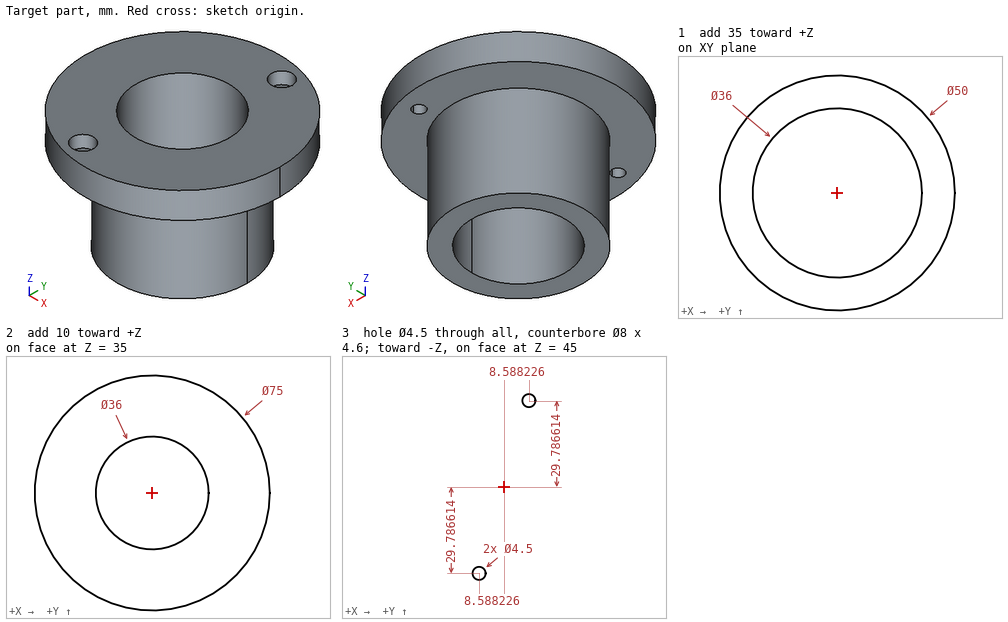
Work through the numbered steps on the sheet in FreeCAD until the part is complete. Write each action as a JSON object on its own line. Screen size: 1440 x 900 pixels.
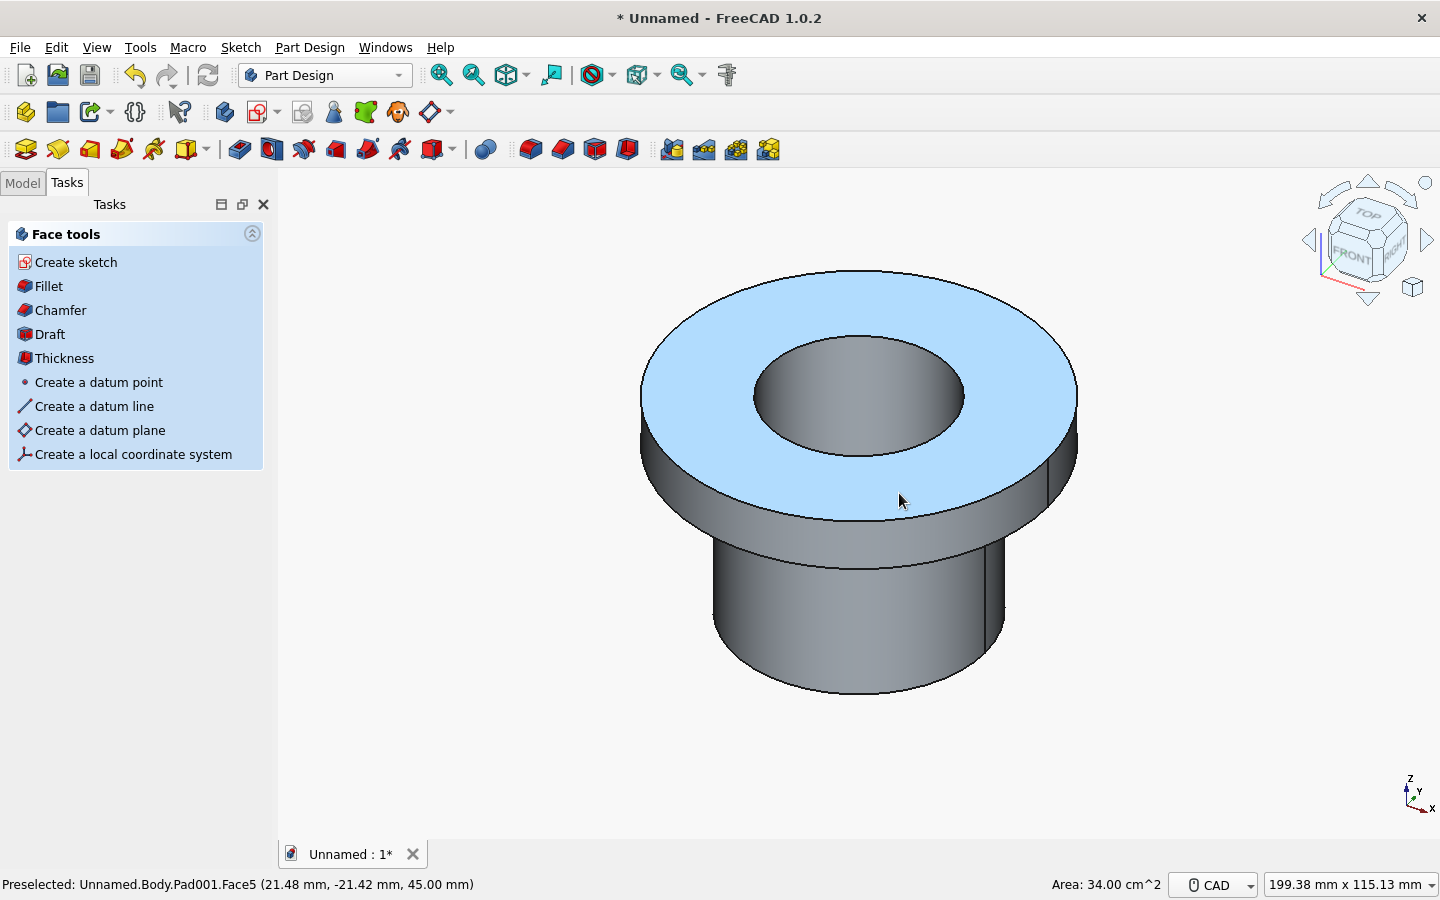
{"action": "left_click", "coordinate": [258, 112]}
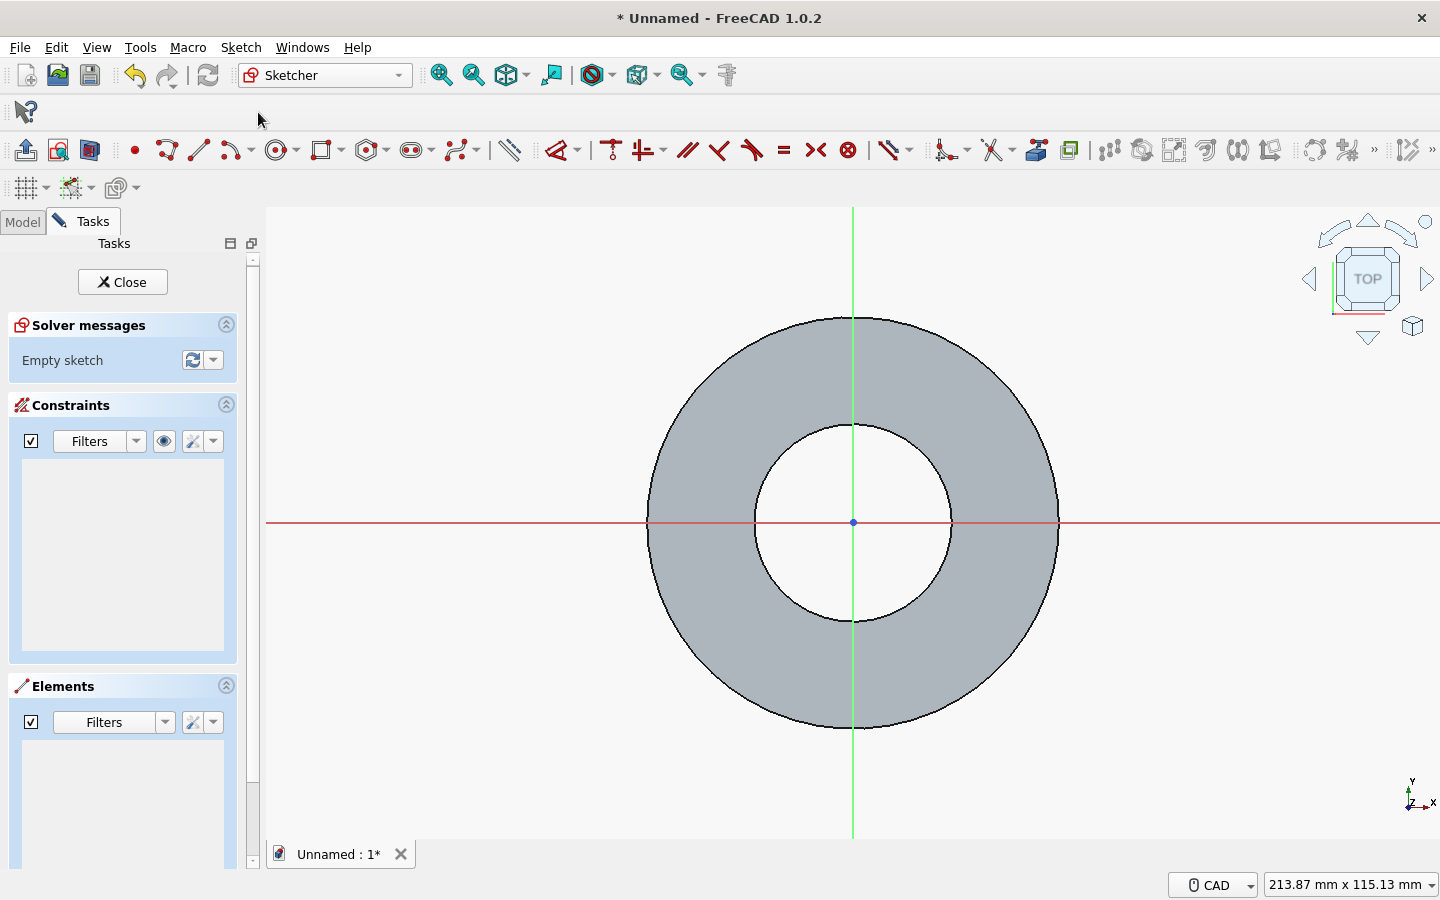
{"action": "key", "text": "g c"}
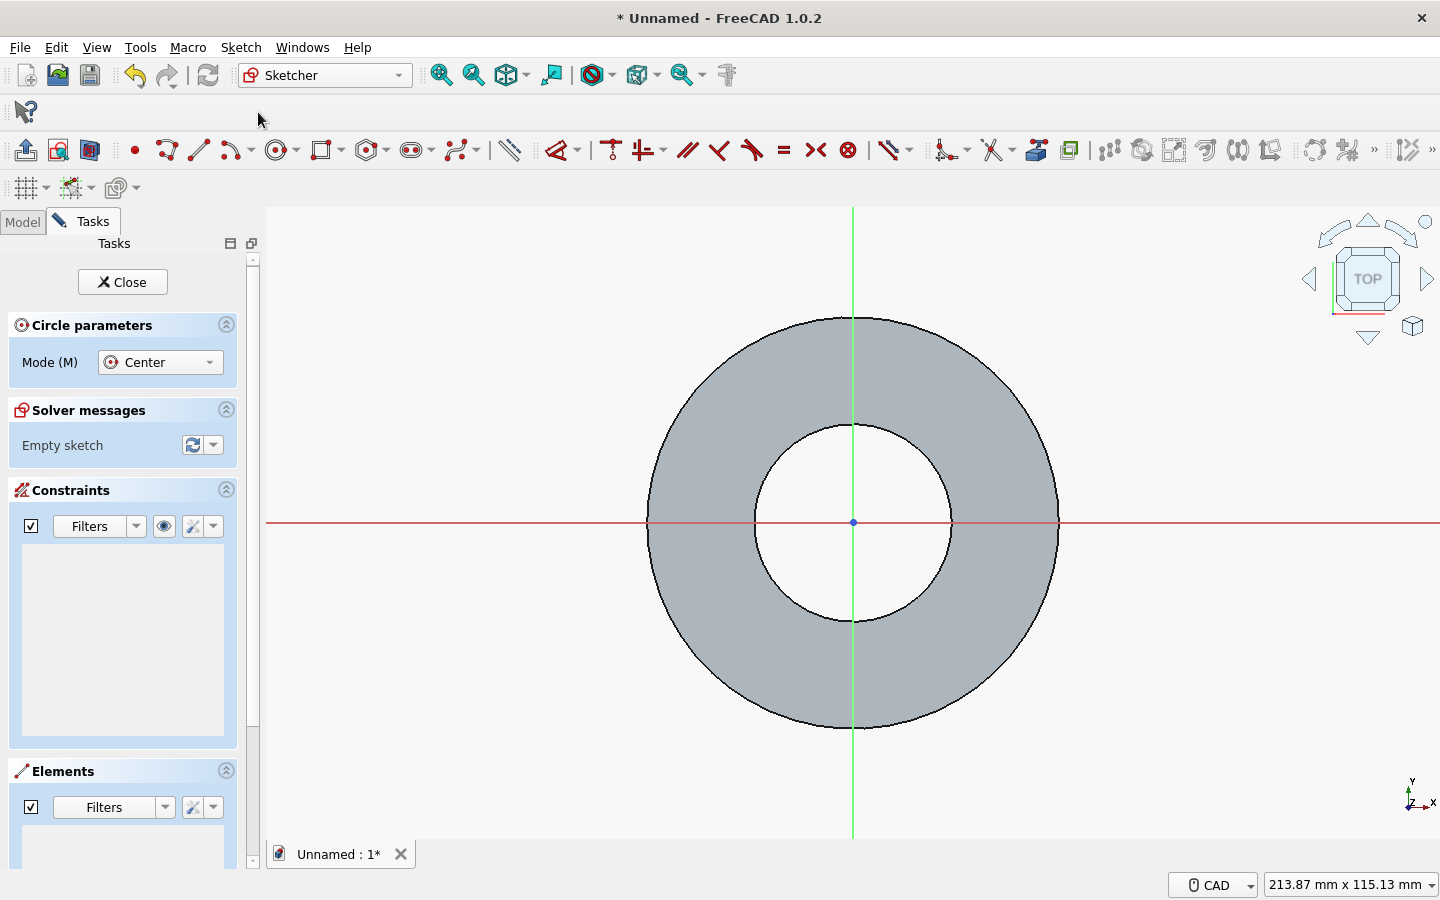
{"action": "scroll", "coordinate": [806, 687], "scroll_direction": "up", "scroll_amount": 4}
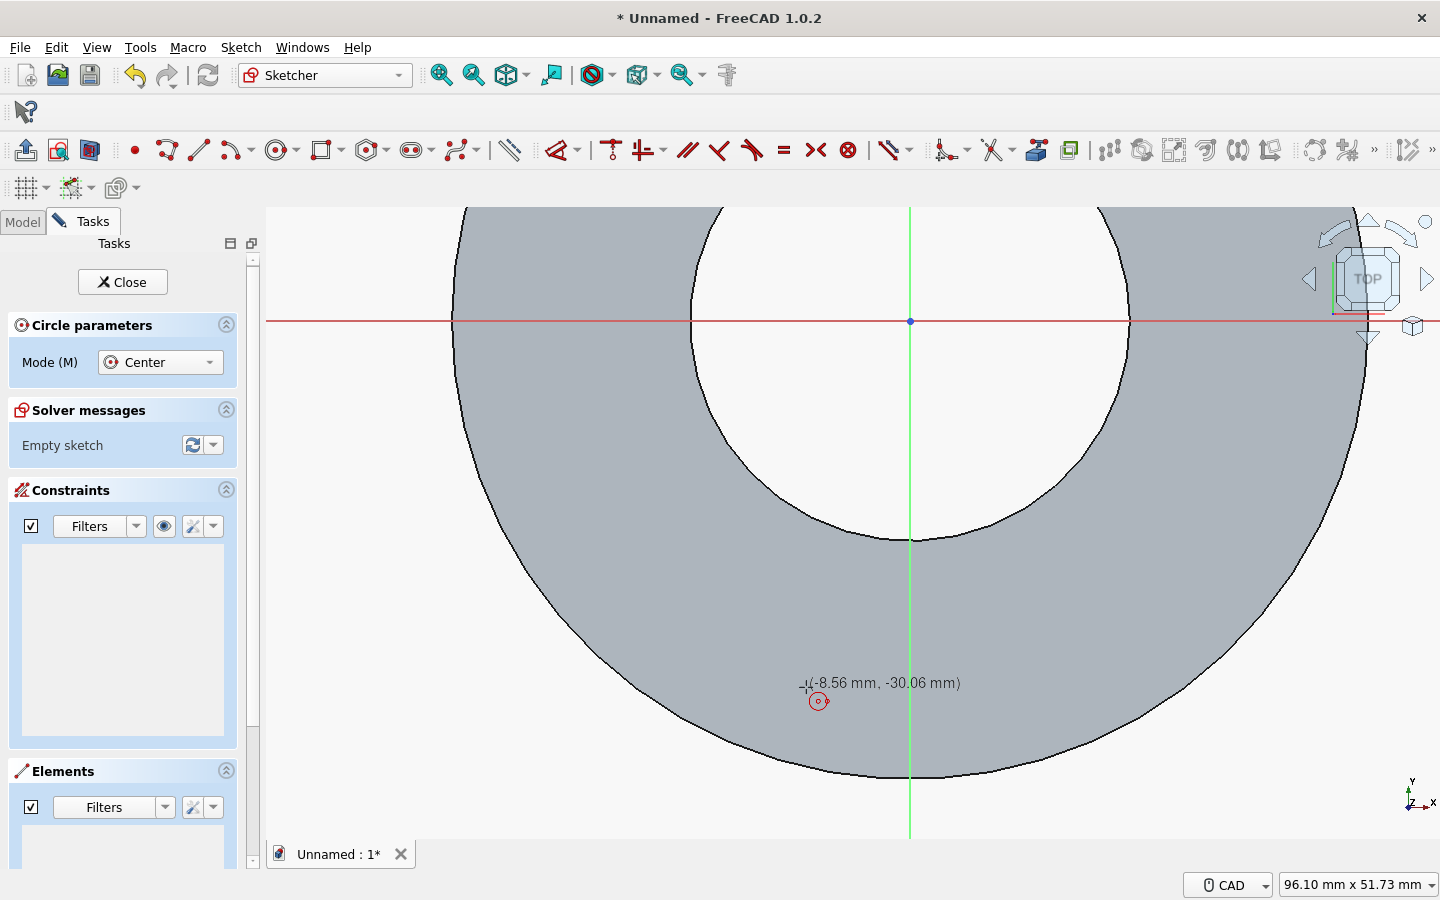
{"action": "left_click", "coordinate": [805, 685]}
{"action": "left_click", "coordinate": [825, 666]}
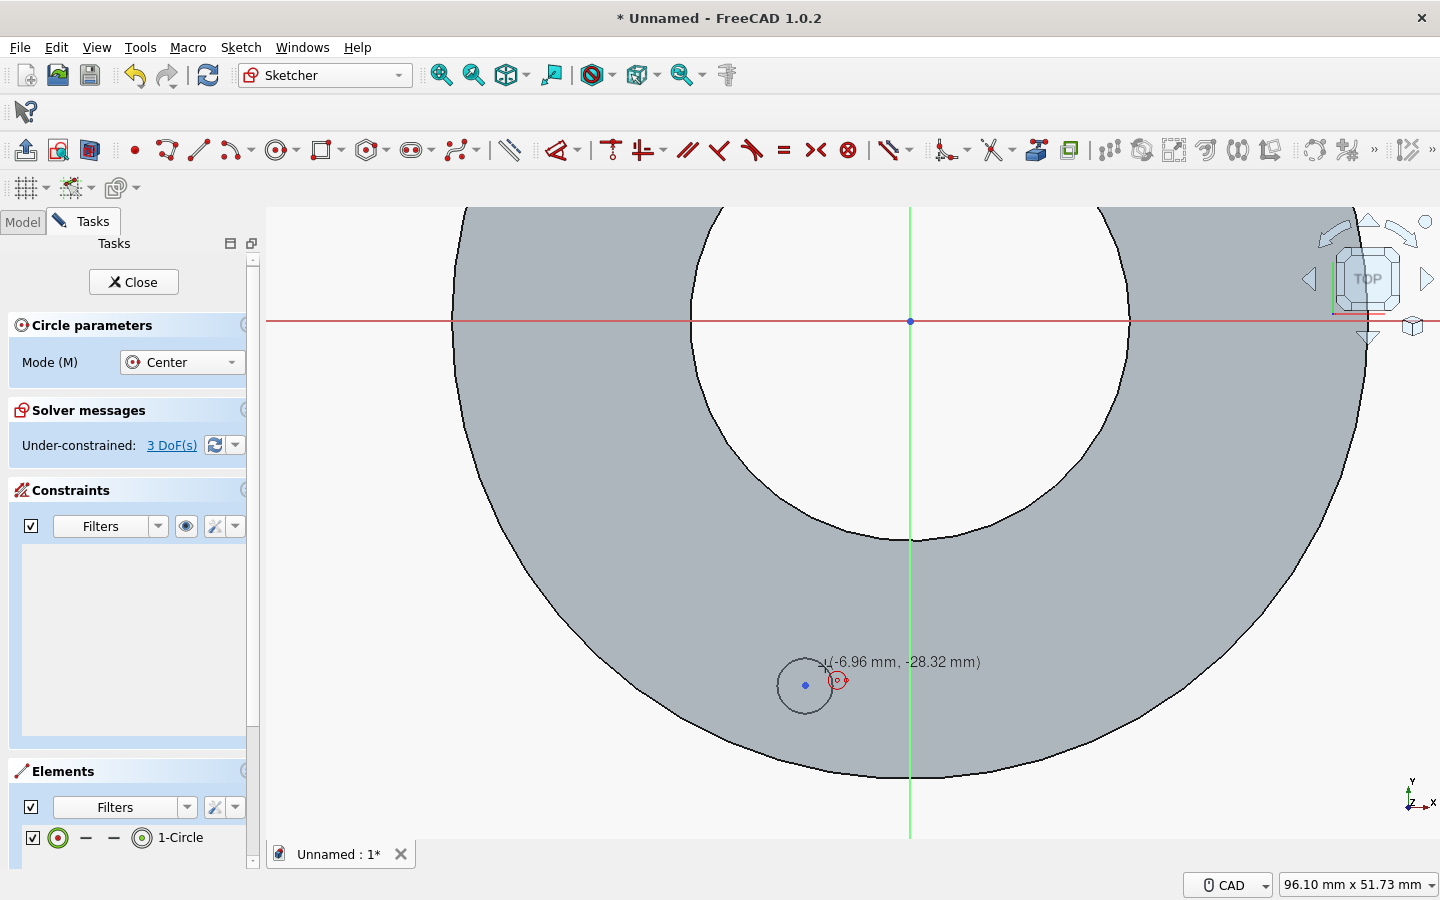
{"action": "scroll", "coordinate": [632, 769], "scroll_direction": "down", "scroll_amount": 3}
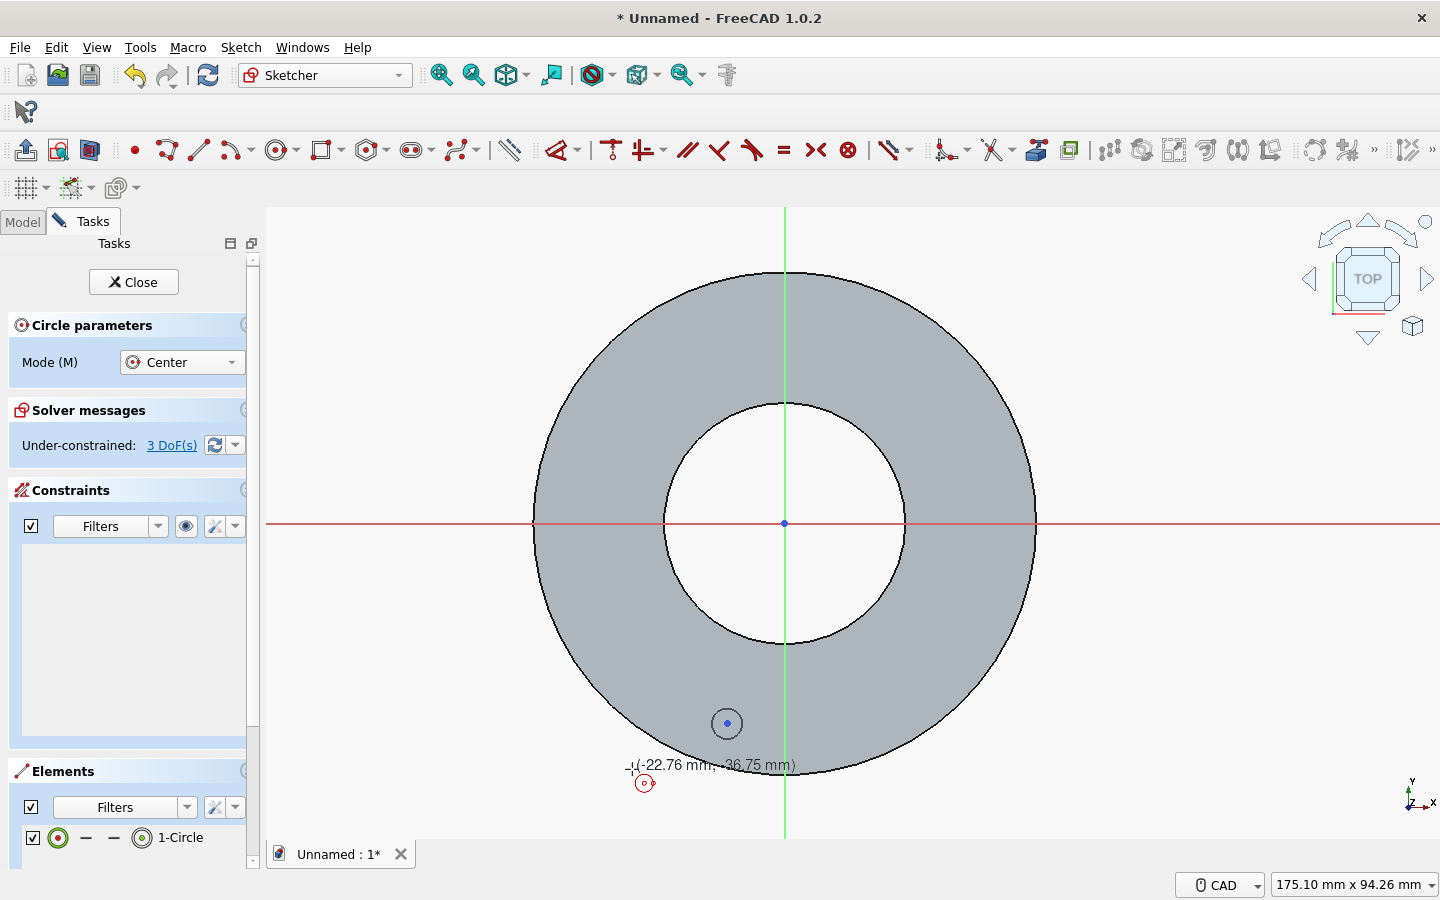
{"action": "scroll", "coordinate": [842, 324], "scroll_direction": "up", "scroll_amount": 3}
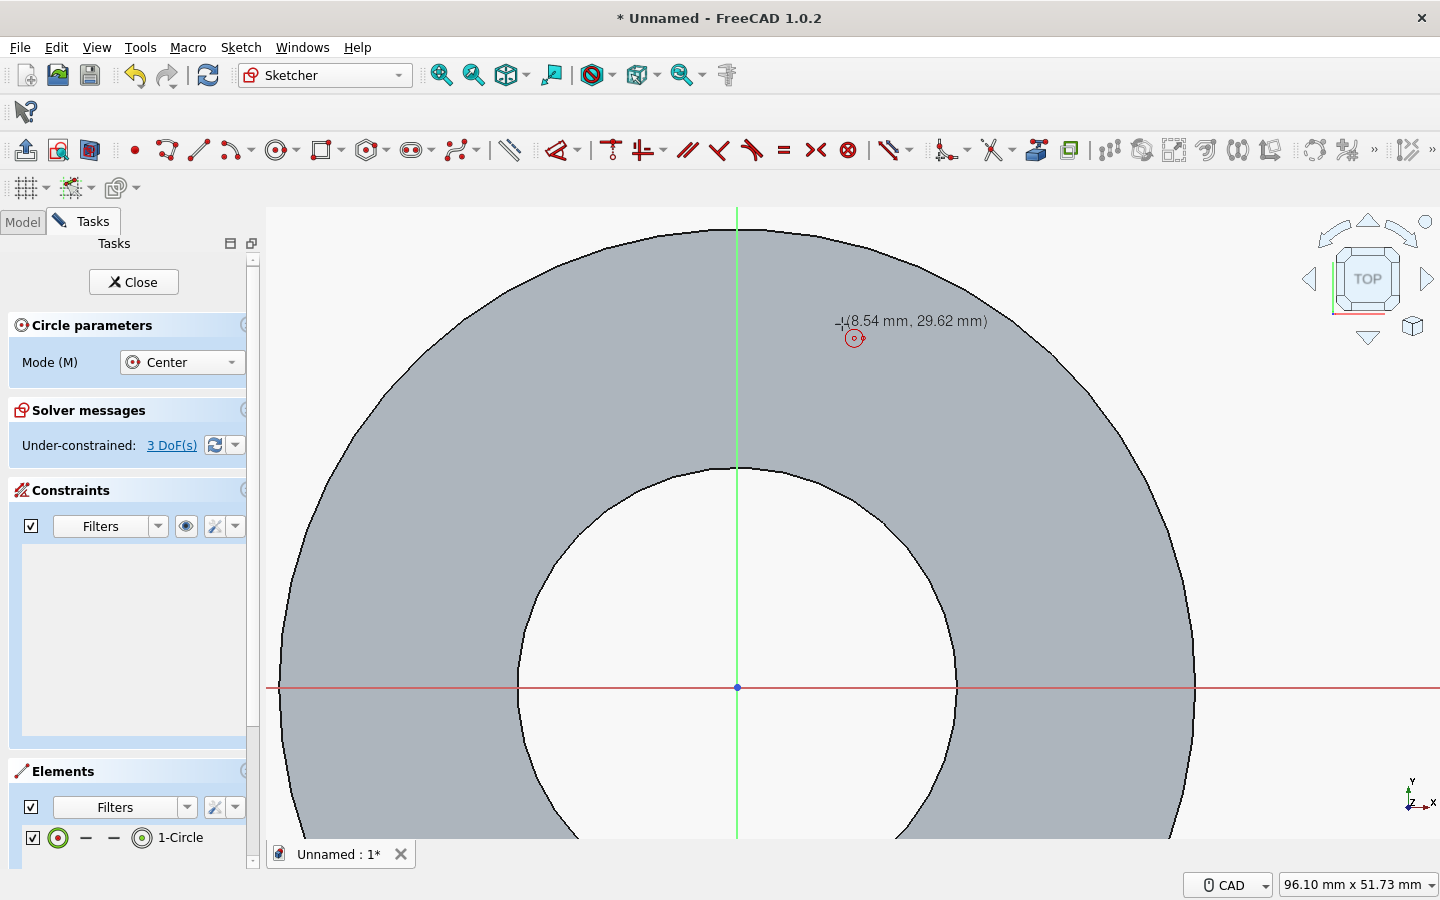
{"action": "left_click", "coordinate": [842, 324]}
{"action": "left_click", "coordinate": [862, 304]}
{"action": "key", "text": "Escape"}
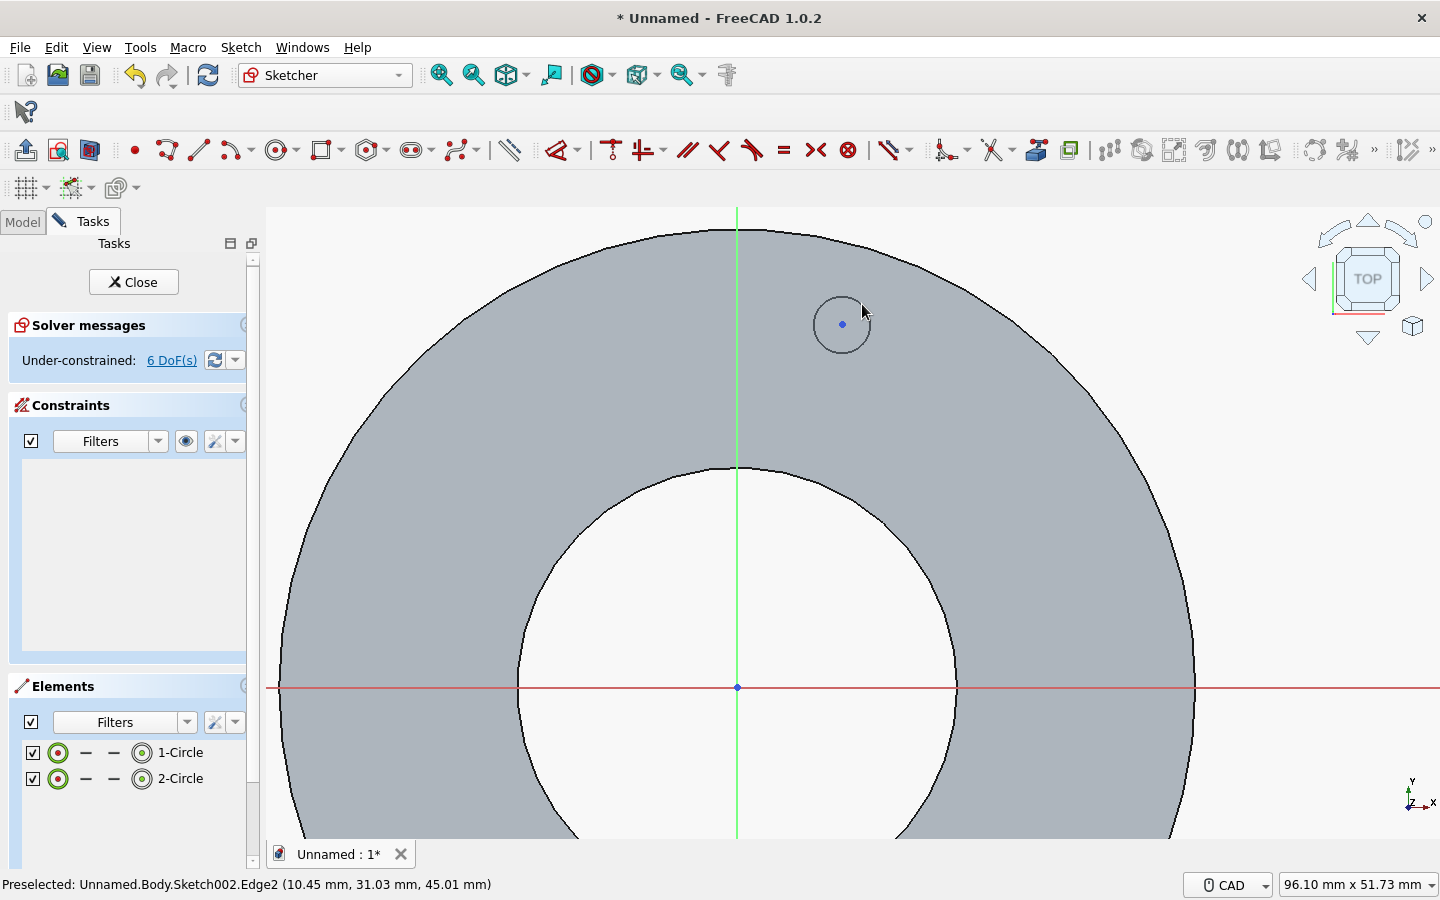
{"action": "scroll", "coordinate": [842, 323], "scroll_direction": "down", "scroll_amount": 3}